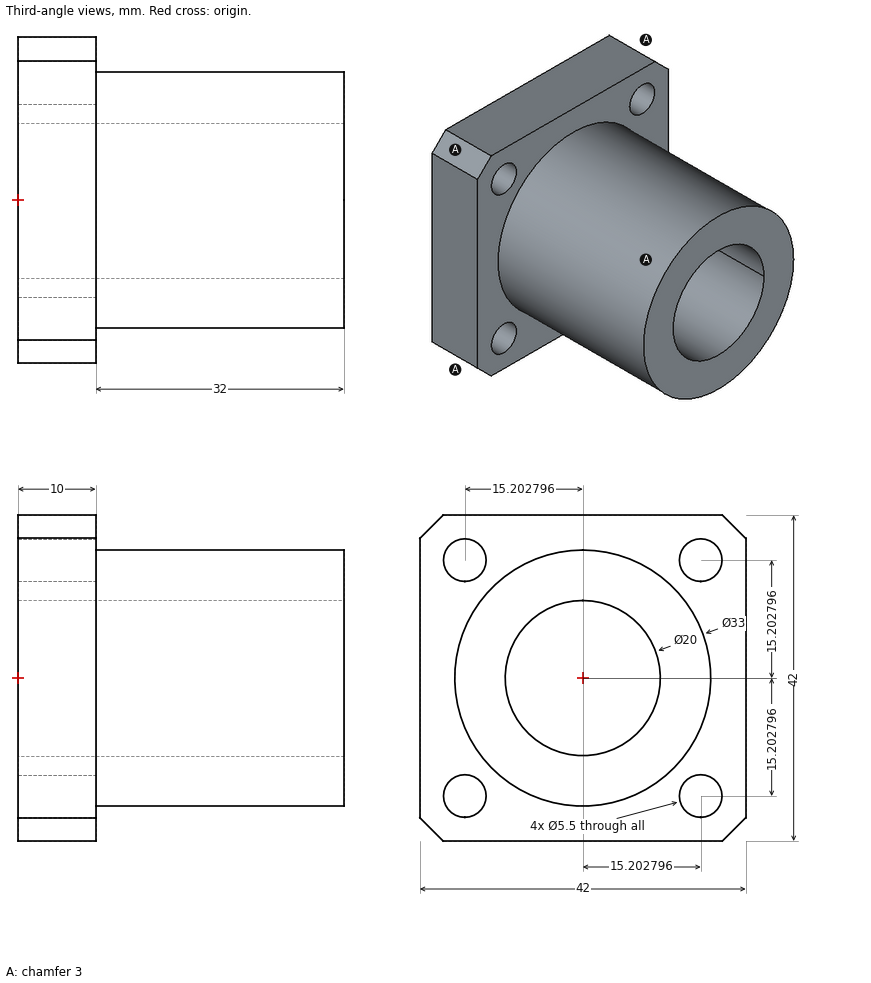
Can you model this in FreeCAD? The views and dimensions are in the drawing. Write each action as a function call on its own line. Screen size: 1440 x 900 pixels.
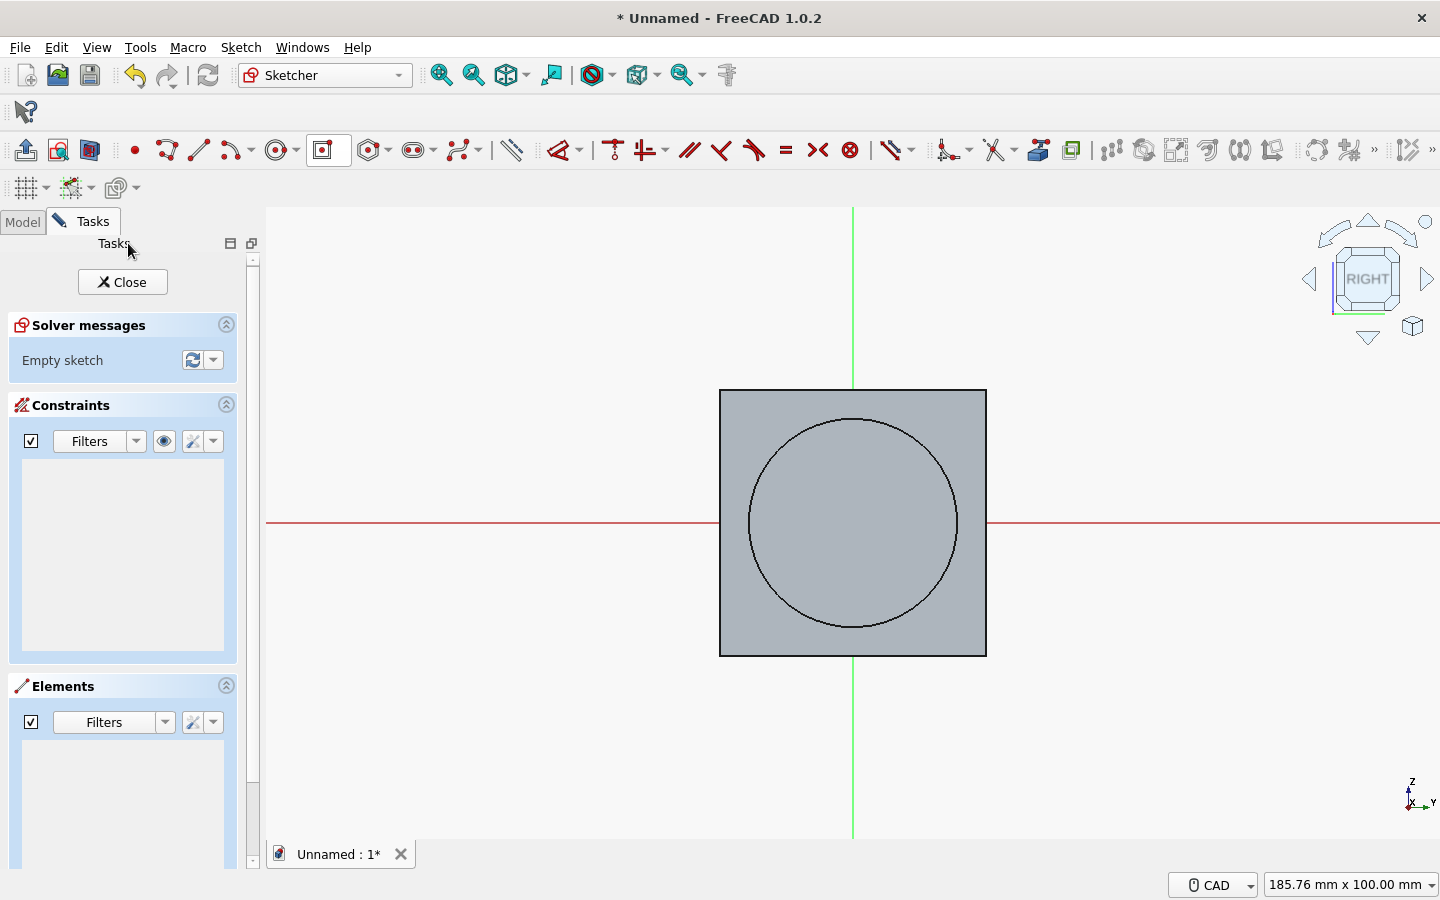
click(90, 150)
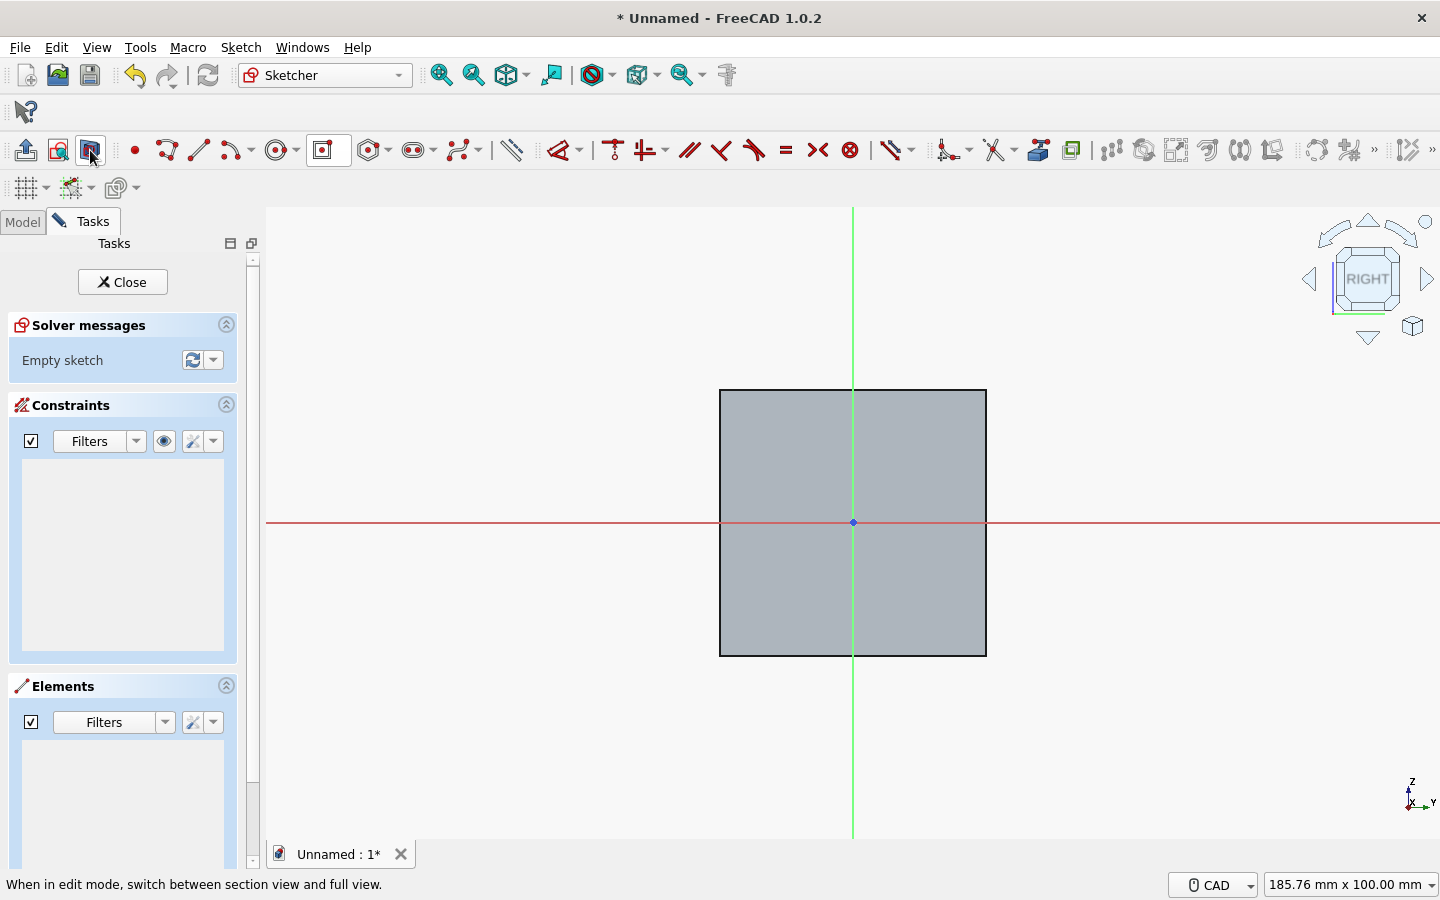
scroll(936, 523, up, 3)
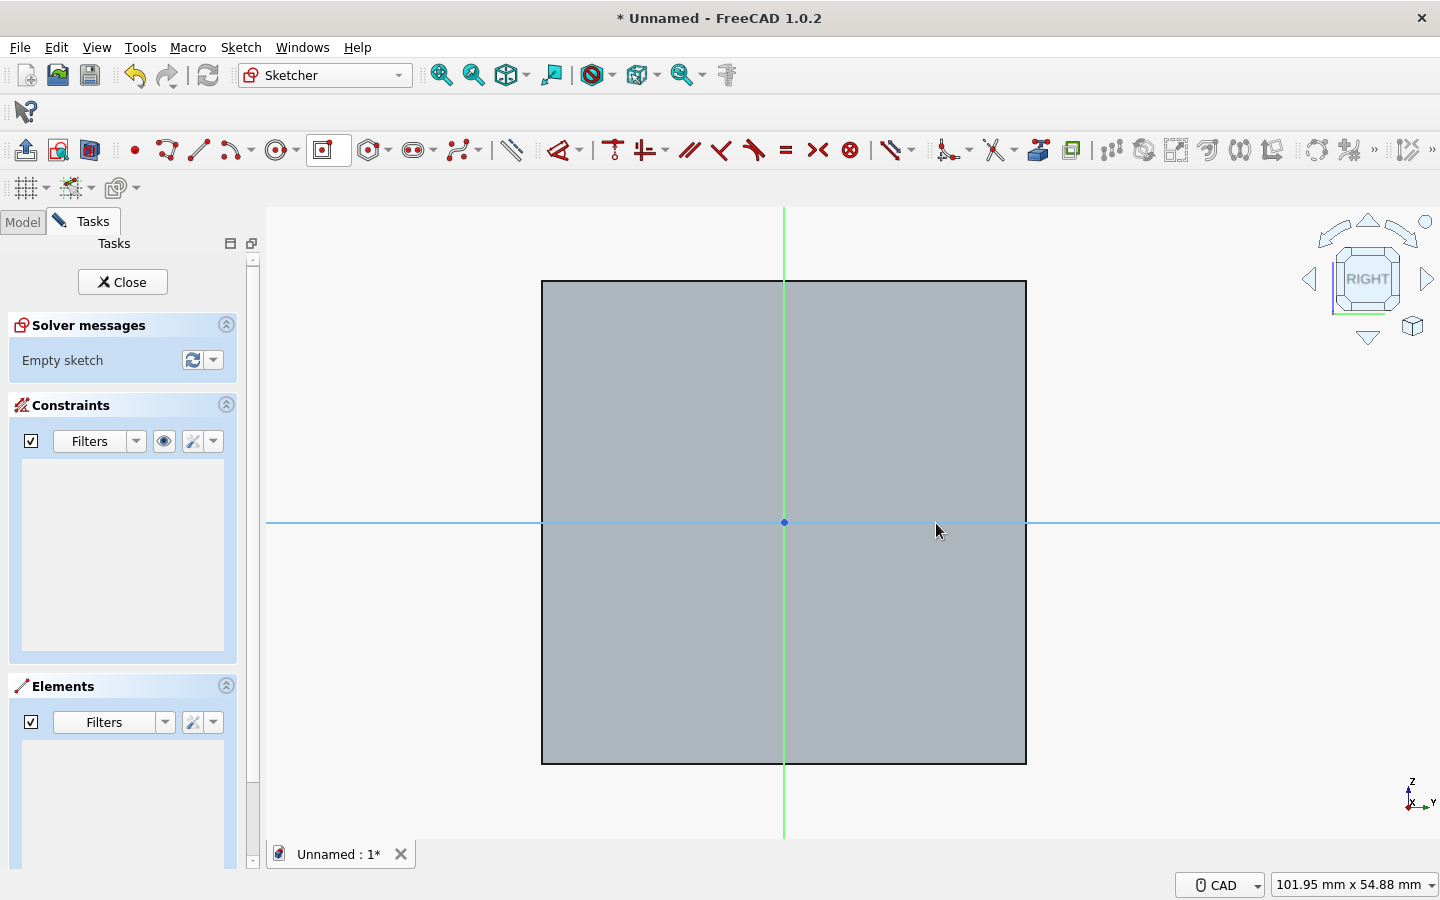
click(276, 150)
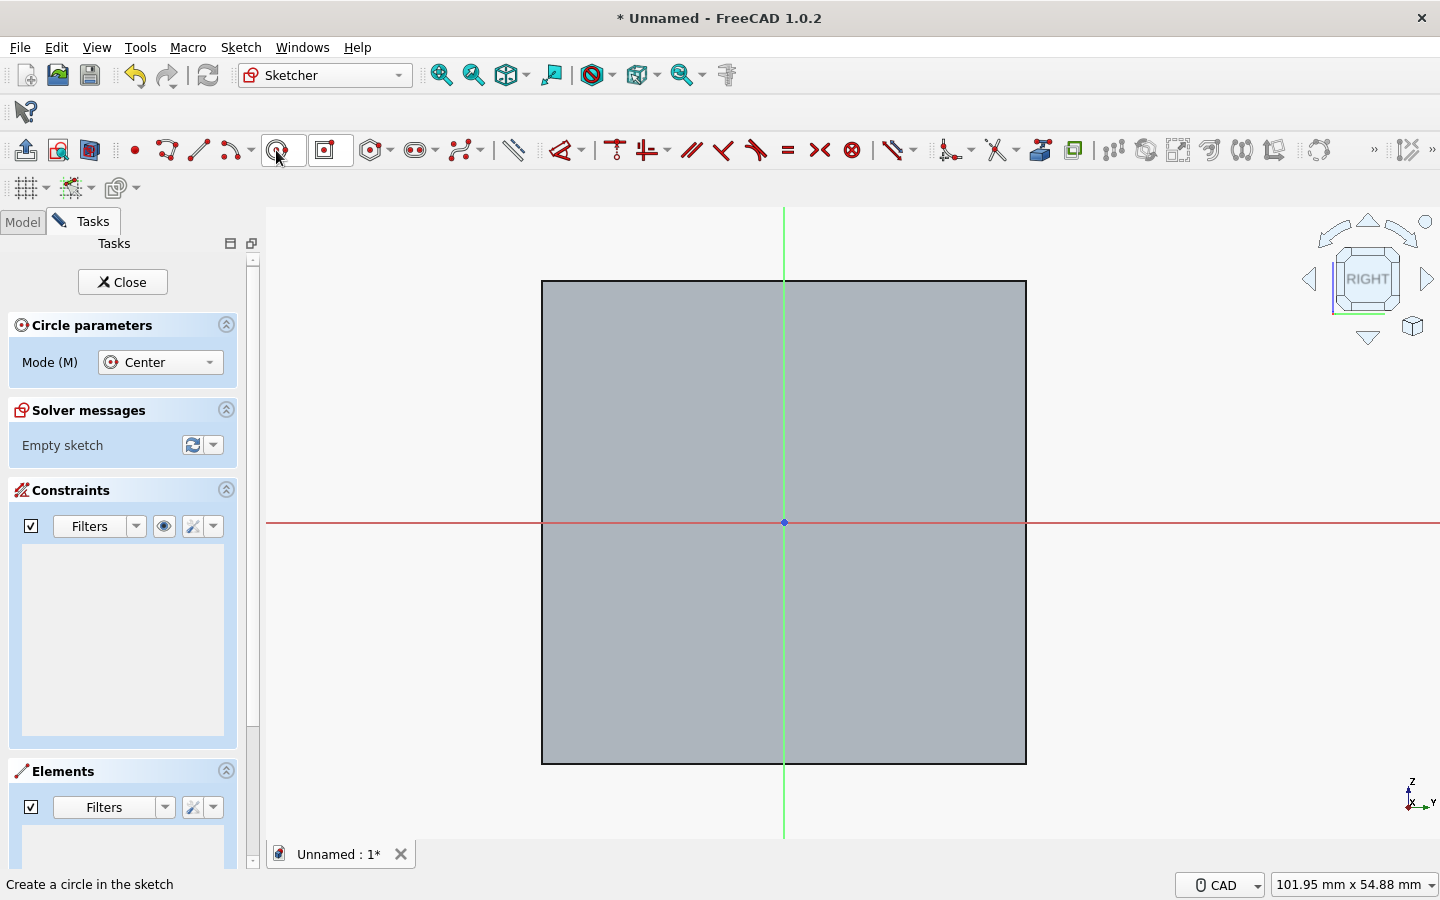
click(959, 698)
click(982, 675)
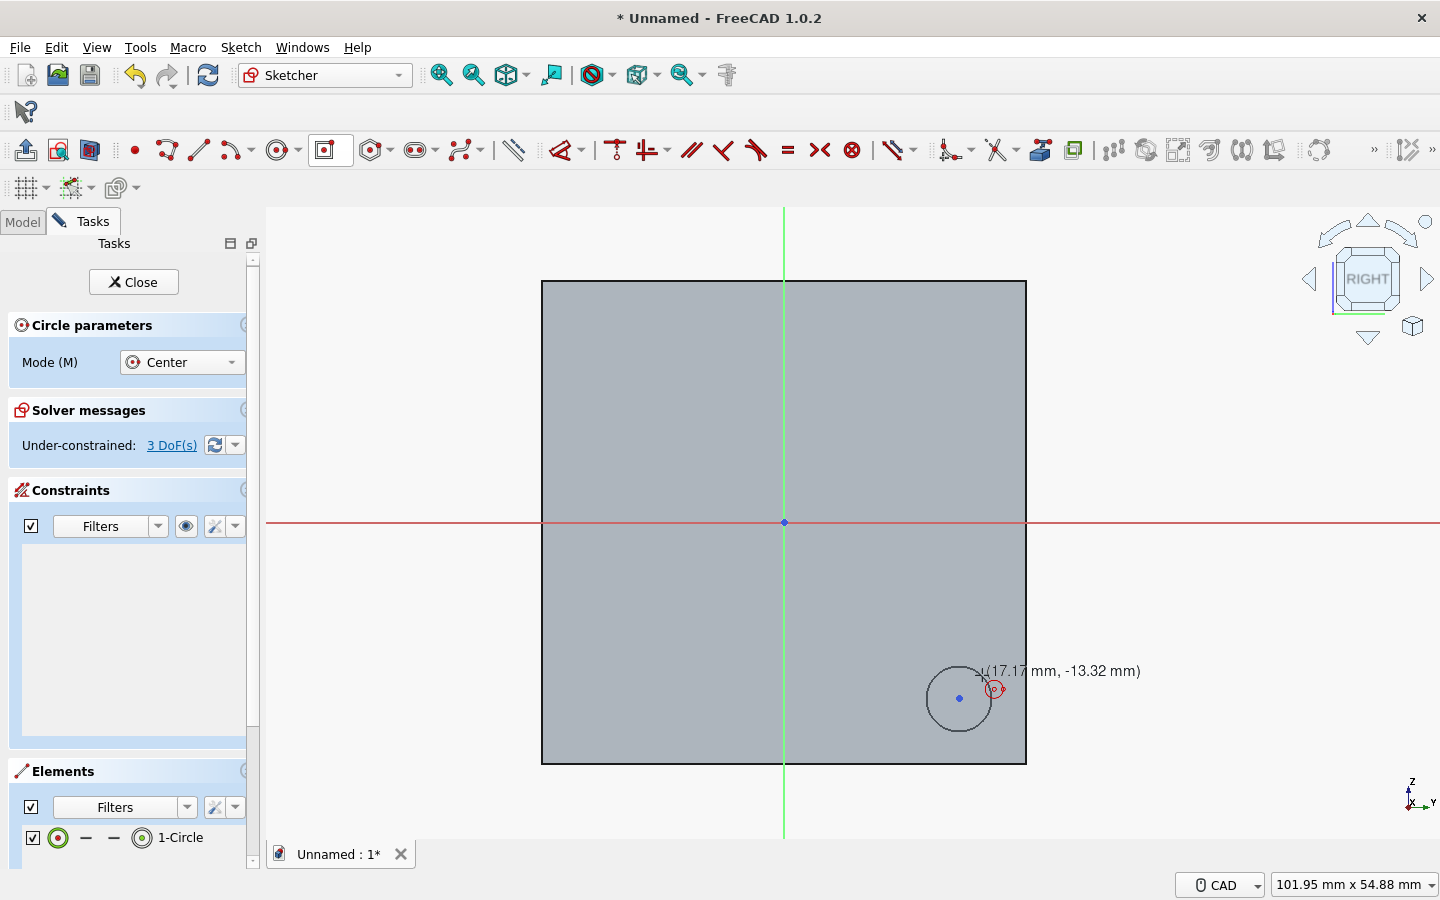
click(959, 348)
click(982, 325)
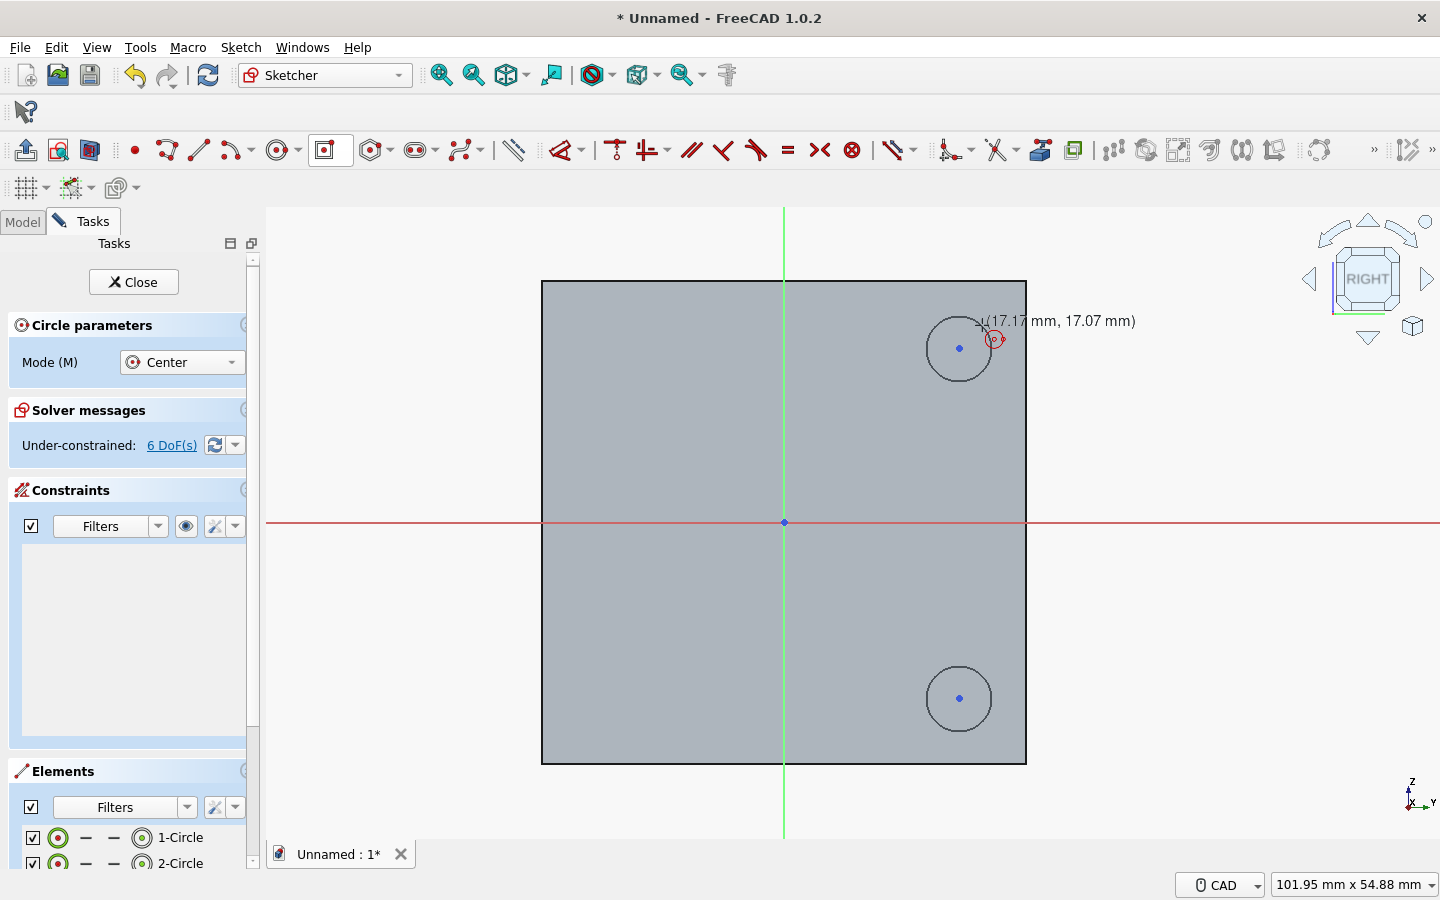
click(609, 348)
click(632, 325)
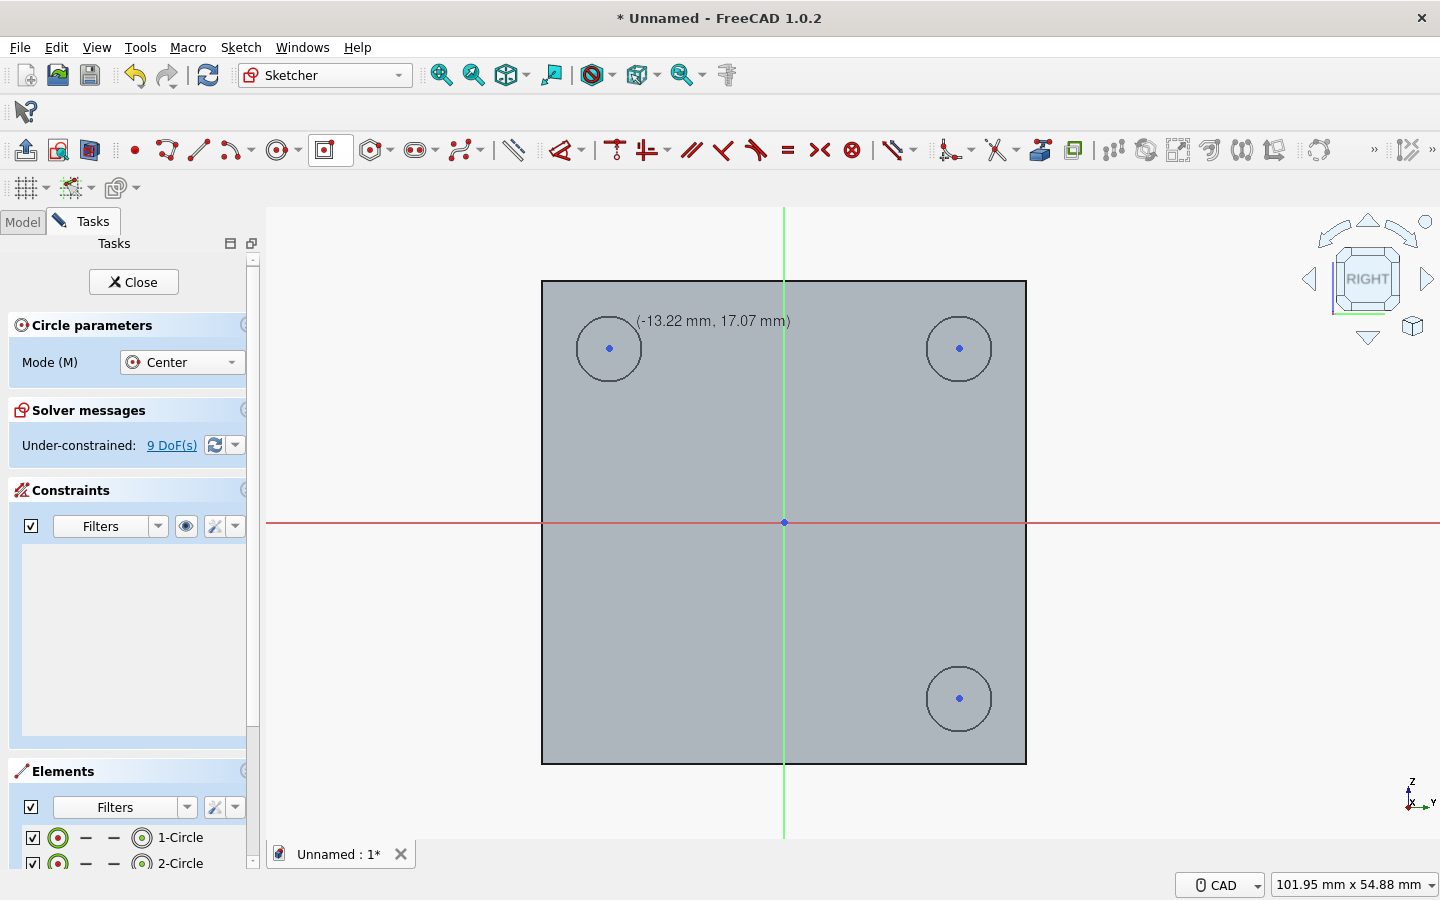
click(609, 698)
click(632, 675)
key(Escape)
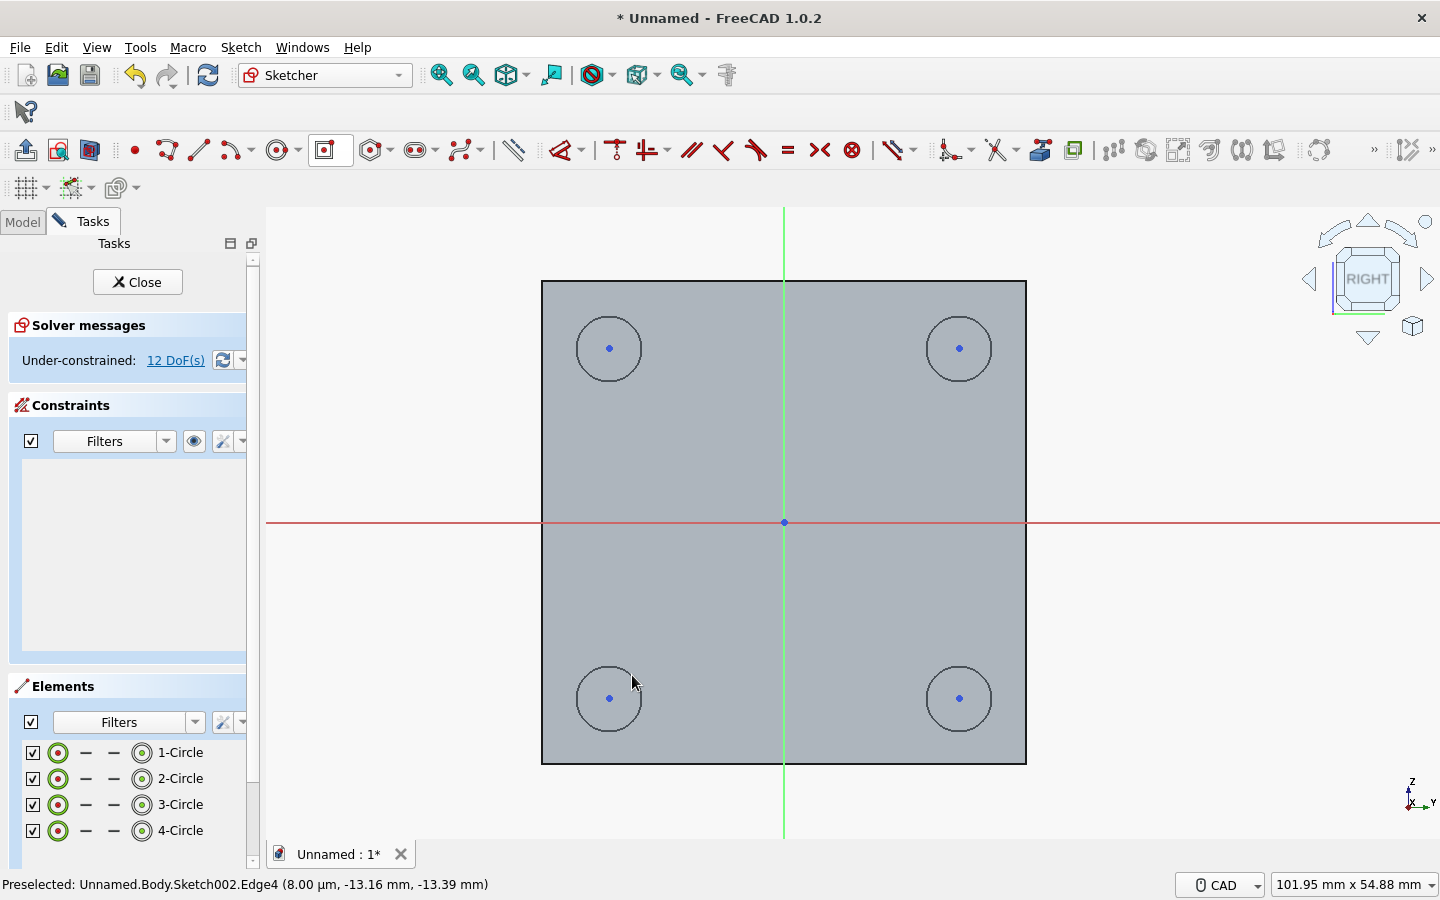
click(982, 676)